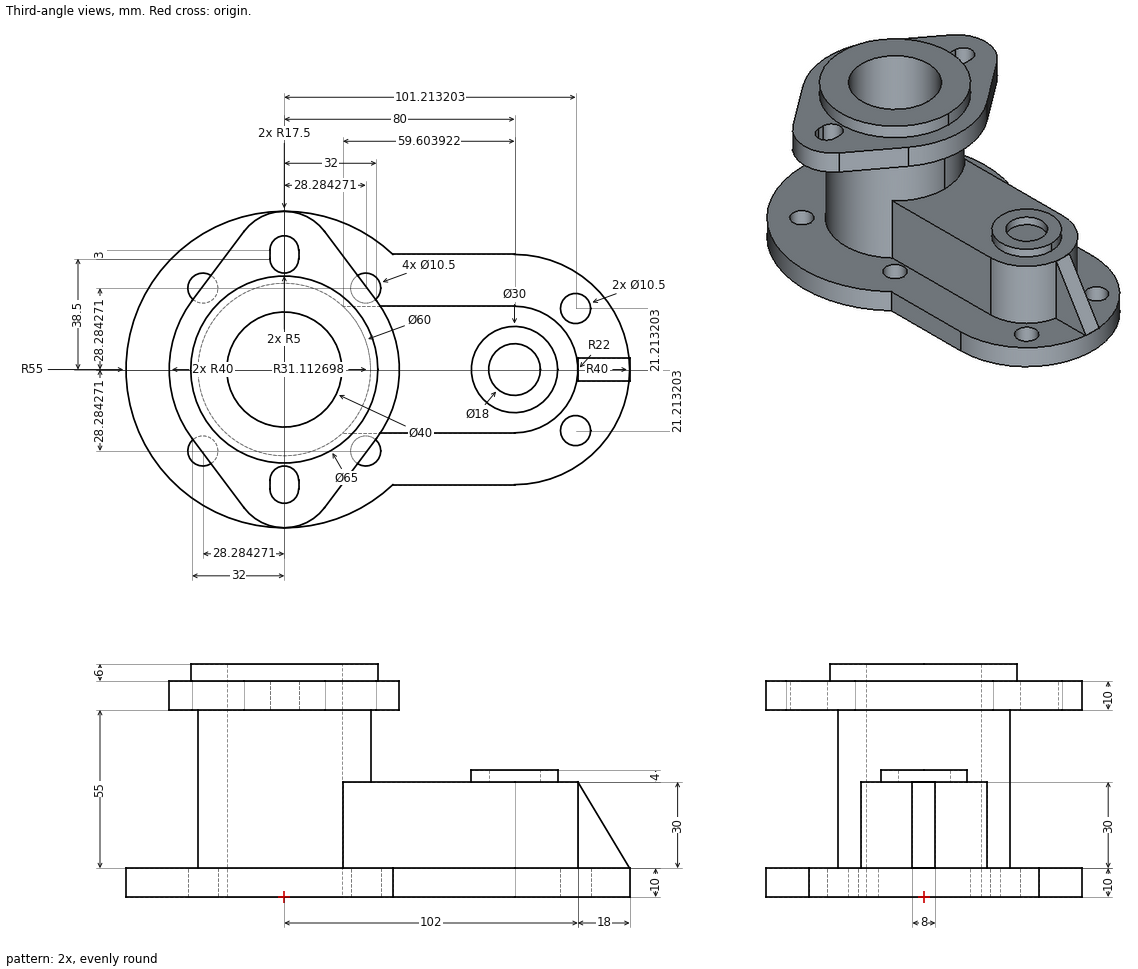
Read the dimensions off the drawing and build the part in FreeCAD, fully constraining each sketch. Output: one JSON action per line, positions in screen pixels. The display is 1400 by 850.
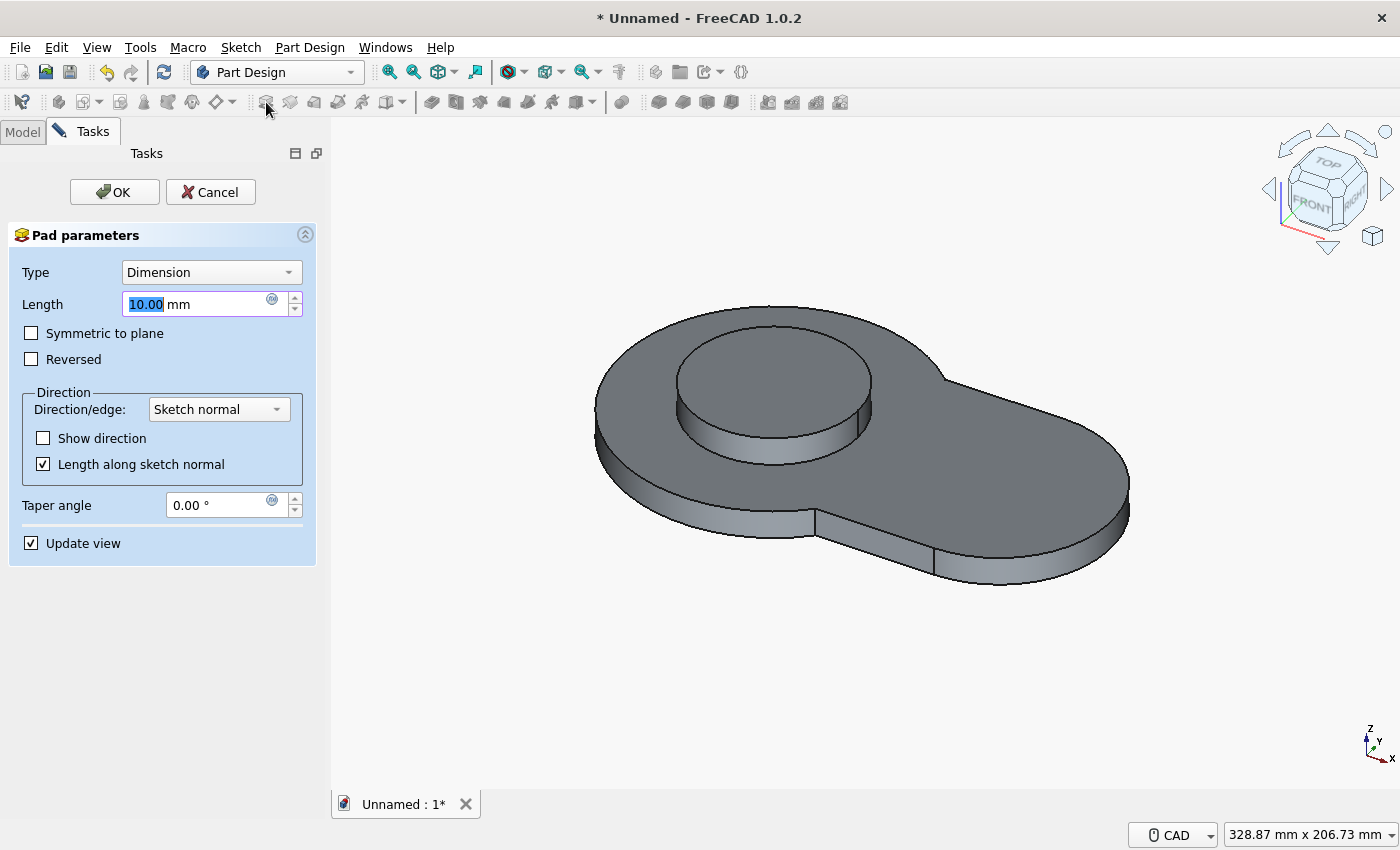
{"action": "type", "text": "55"}
{"action": "key", "text": "Tab"}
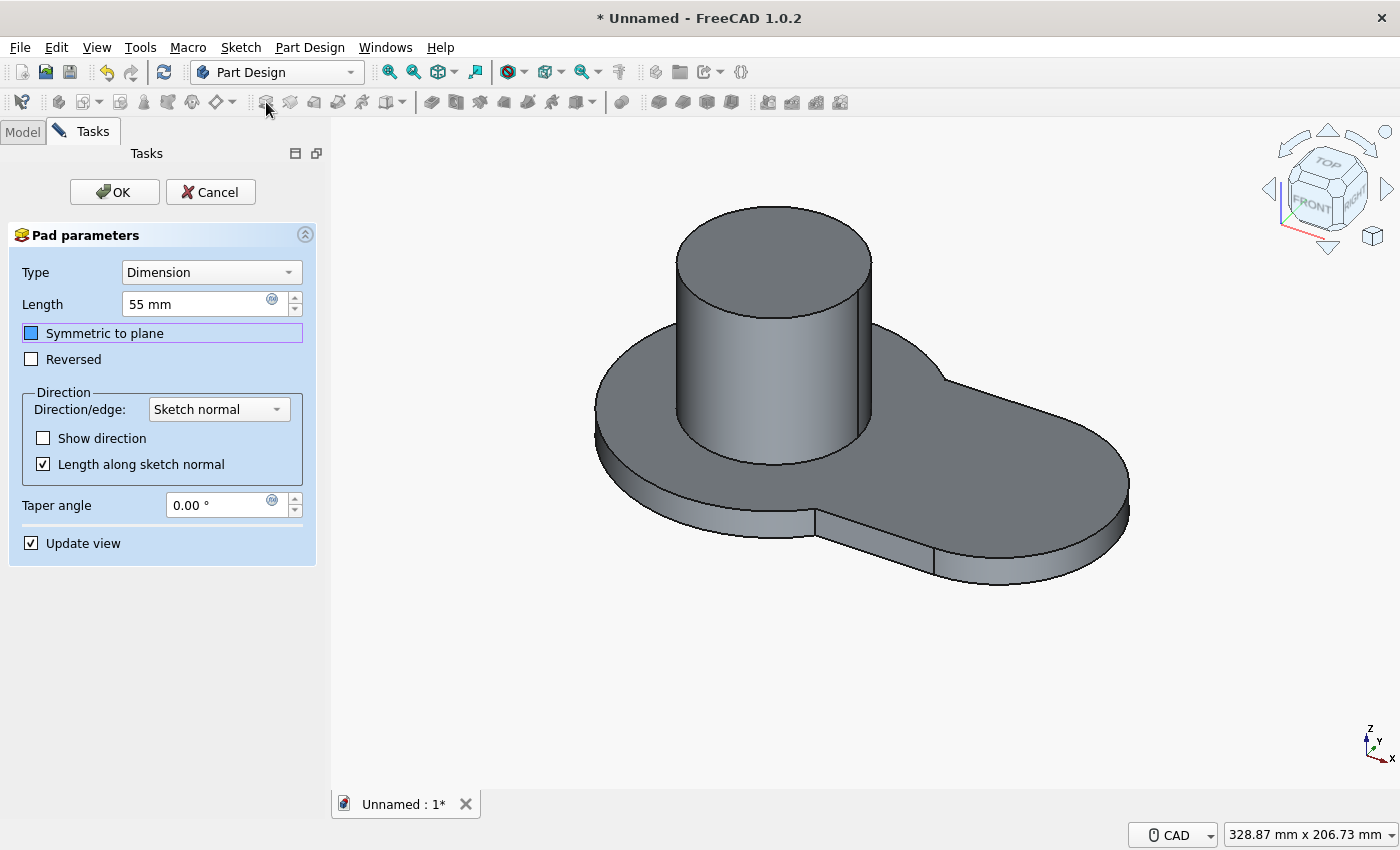
{"action": "left_click", "coordinate": [115, 192]}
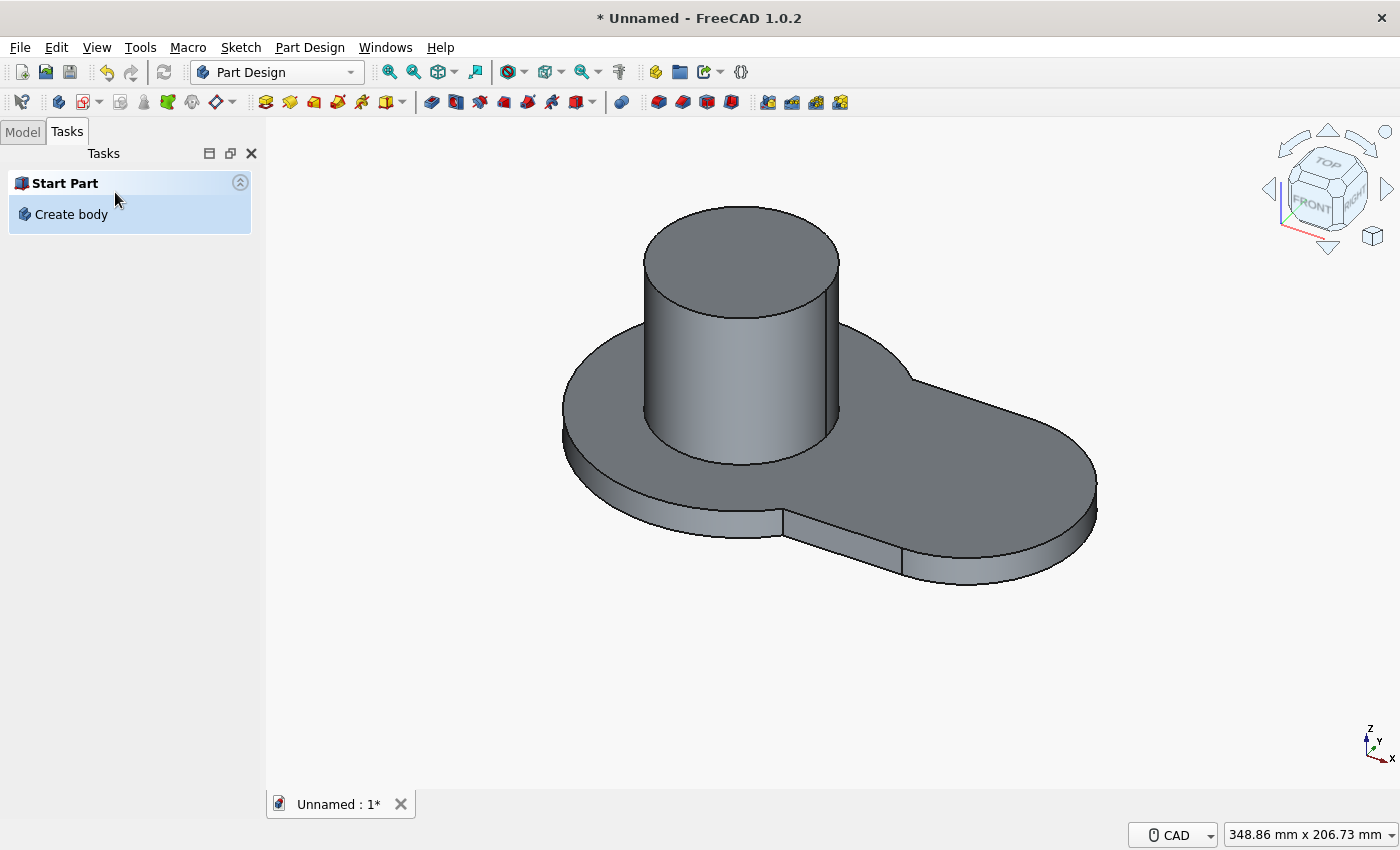
{"action": "left_click", "coordinate": [974, 485]}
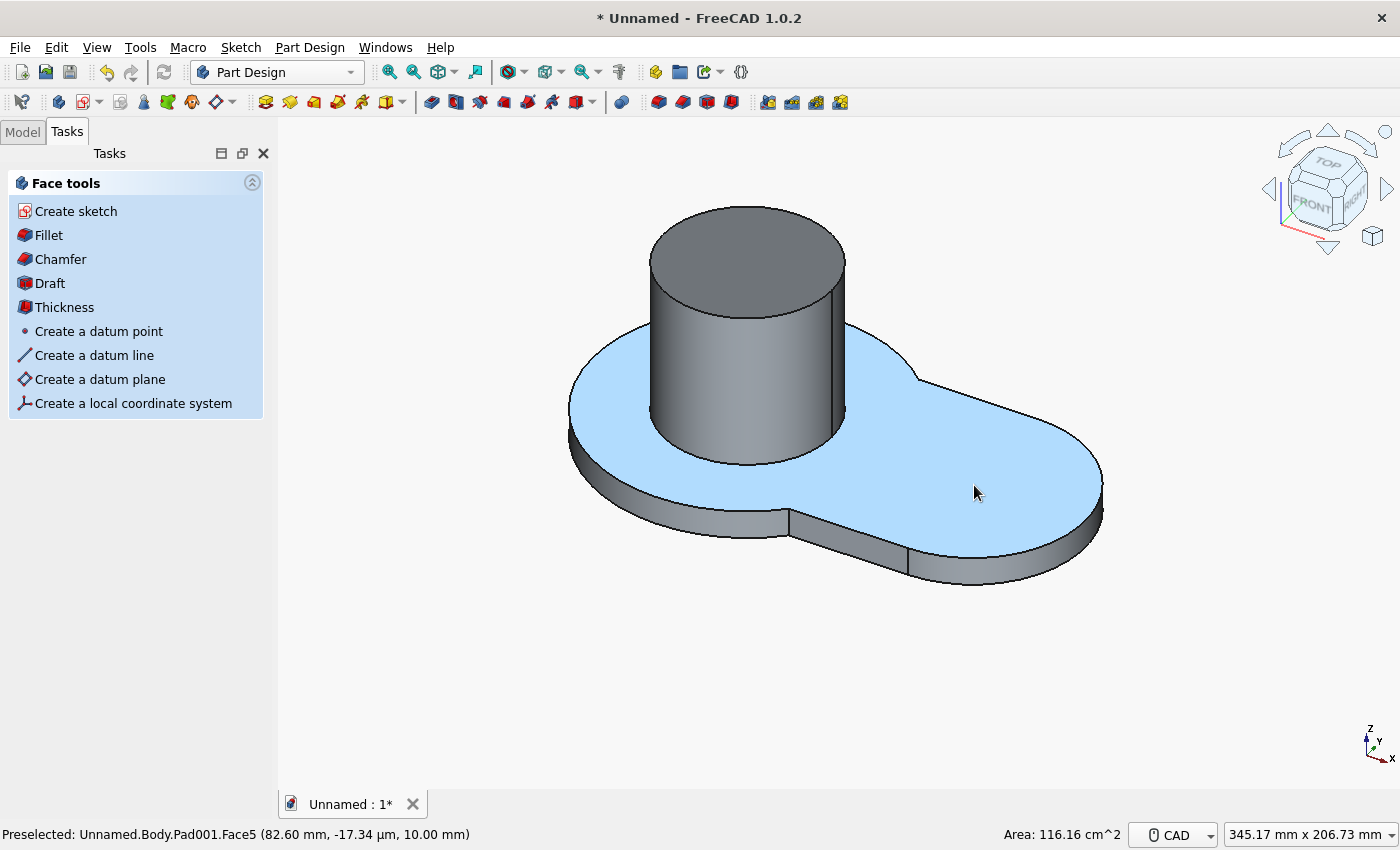
{"action": "left_click", "coordinate": [84, 102]}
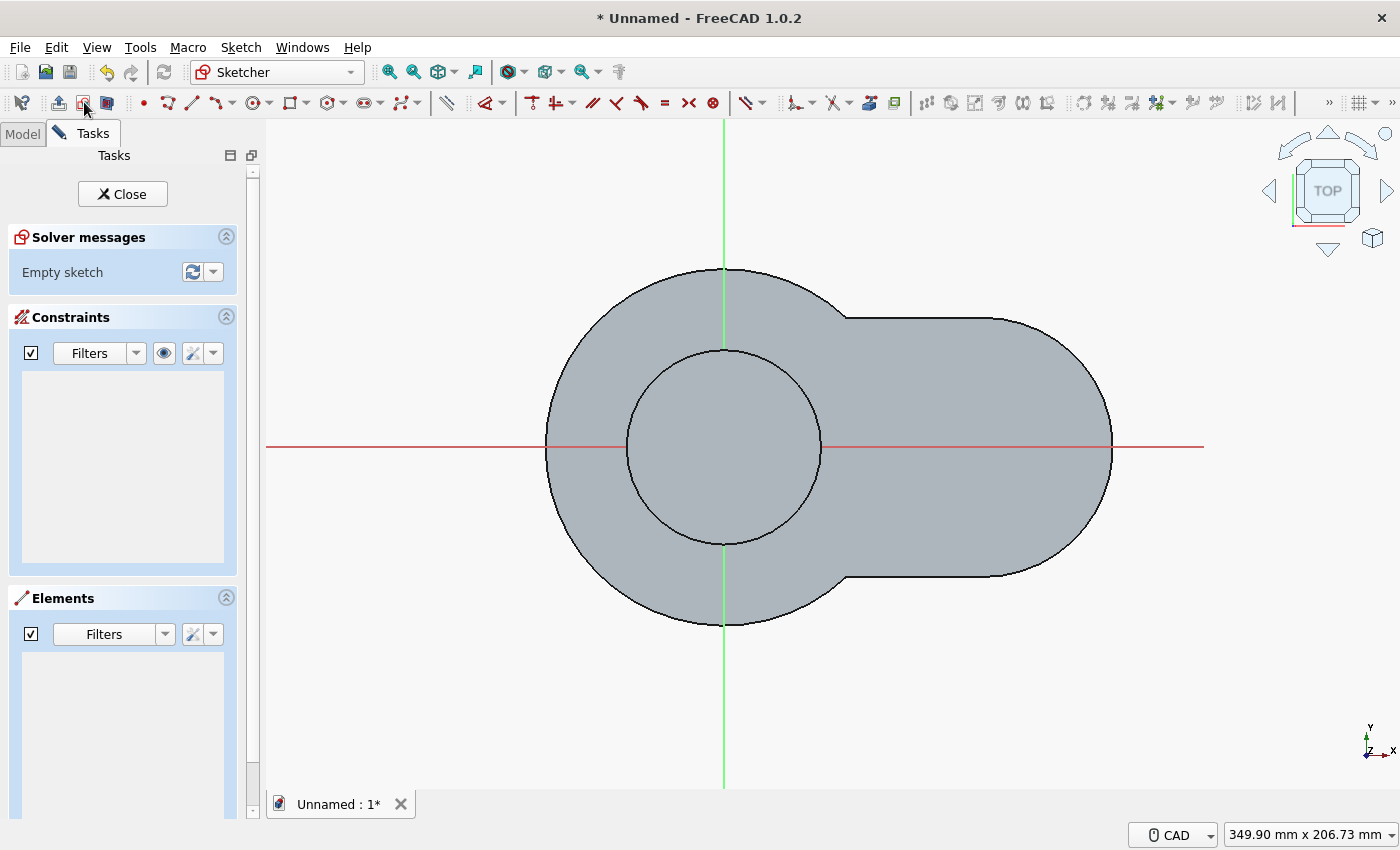
{"action": "key", "text": "q s"}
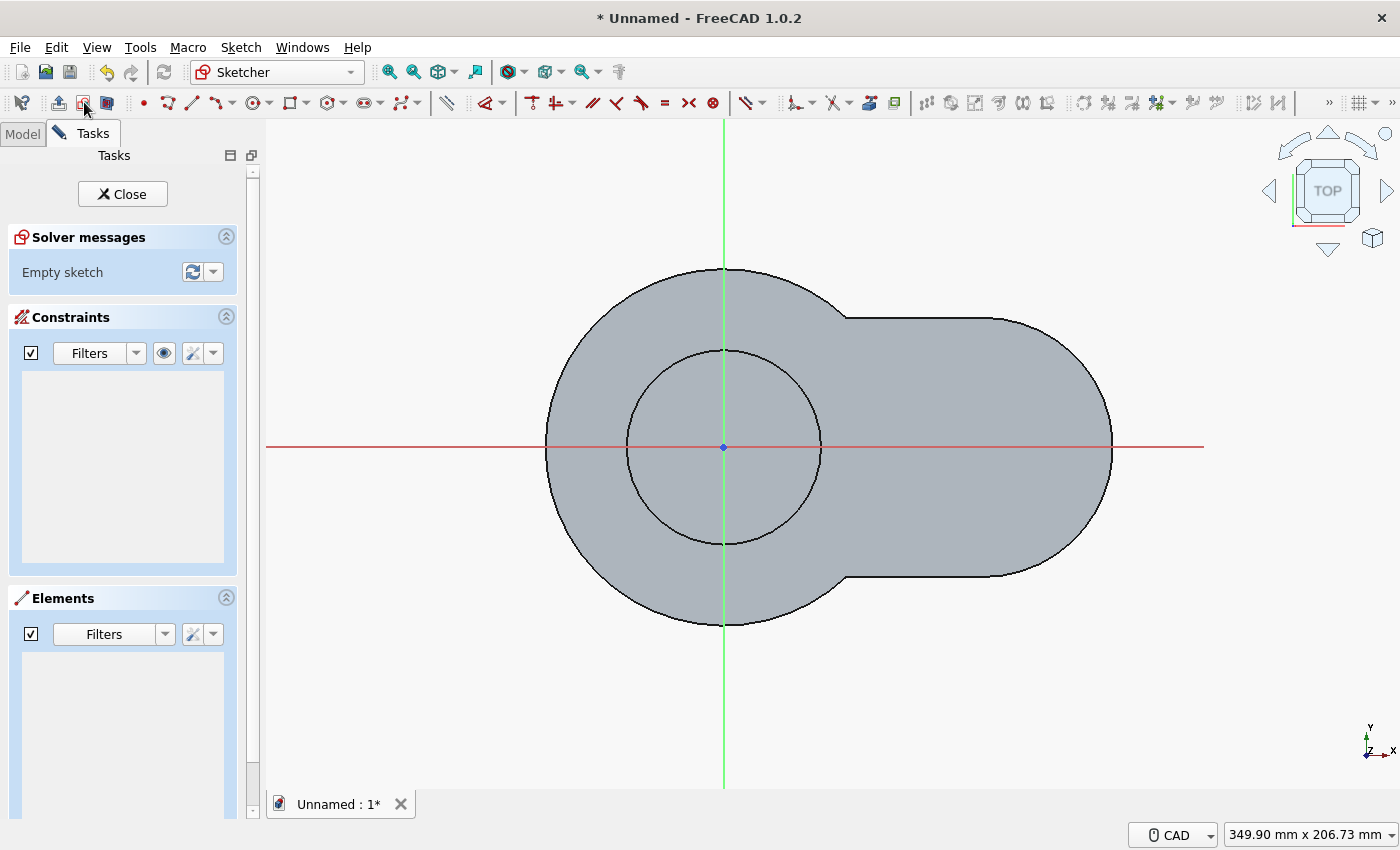
{"action": "scroll", "coordinate": [674, 439], "scroll_direction": "up", "scroll_amount": 3}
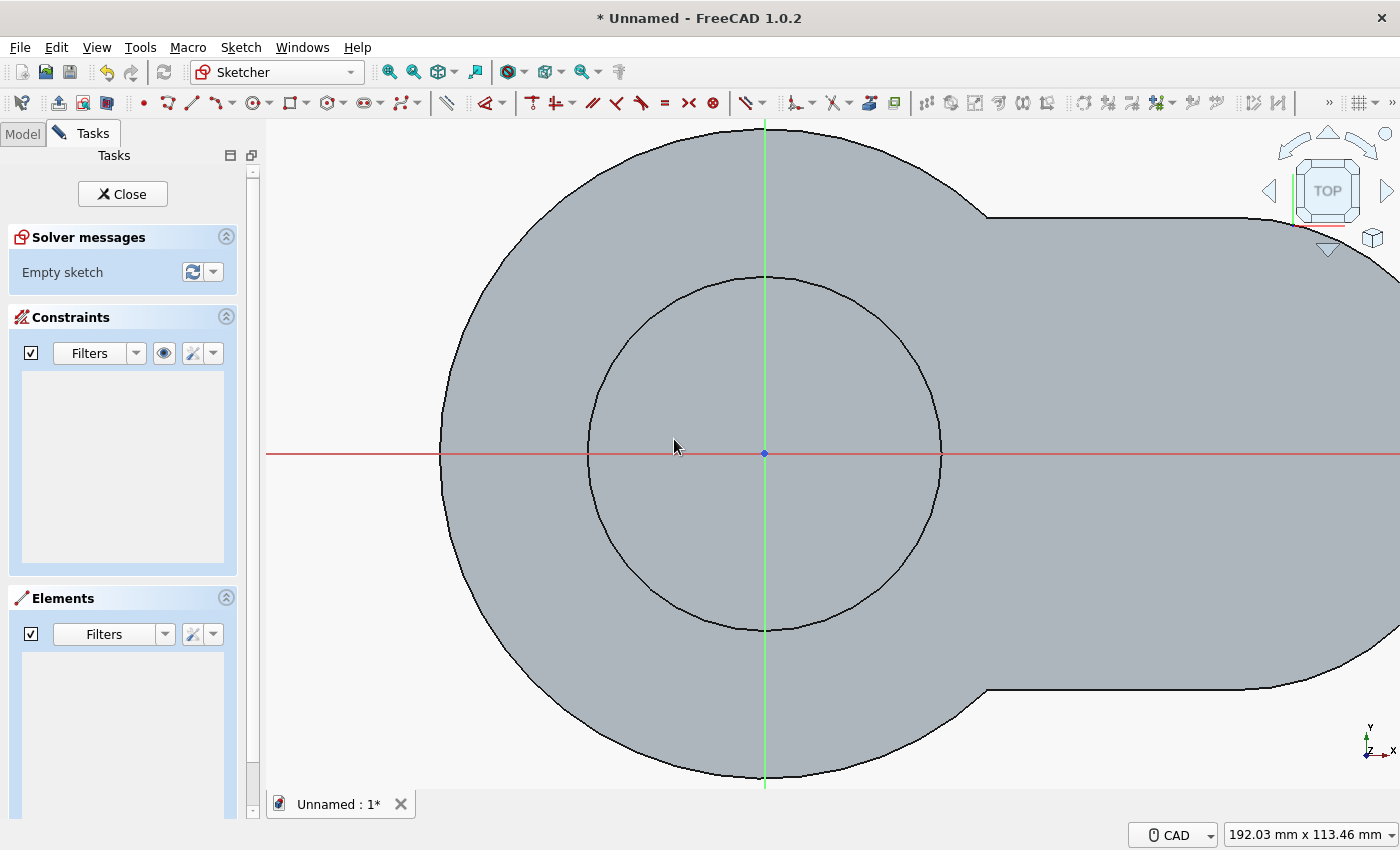
{"action": "key", "text": "g c"}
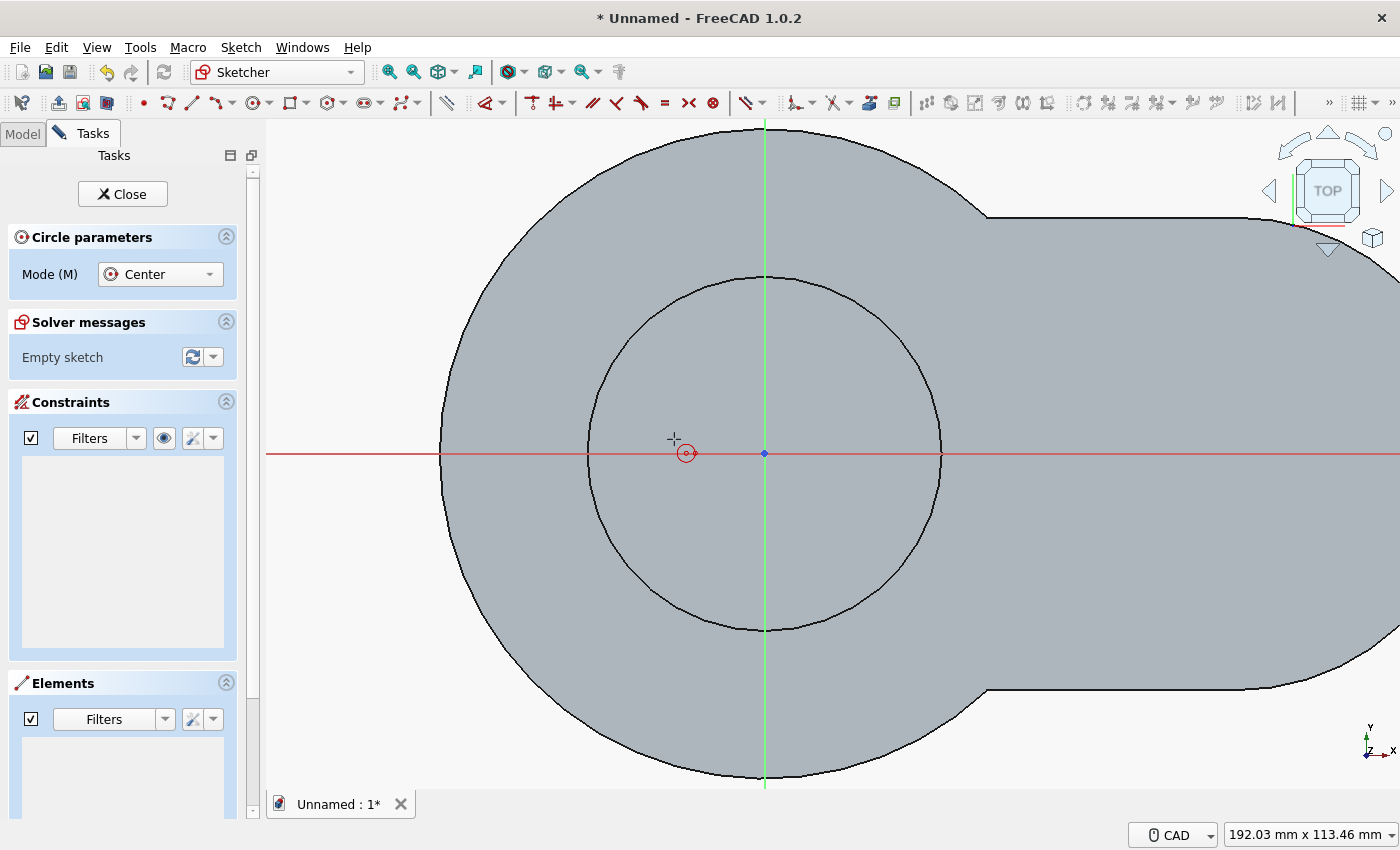
{"action": "left_click", "coordinate": [932, 287]}
{"action": "mouse_move", "coordinate": [953, 265]}